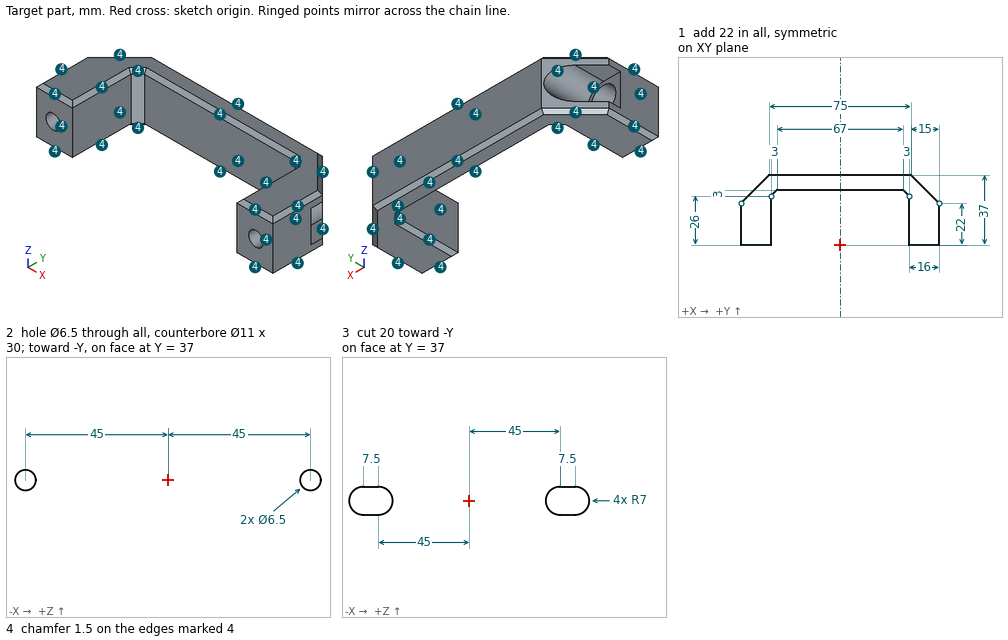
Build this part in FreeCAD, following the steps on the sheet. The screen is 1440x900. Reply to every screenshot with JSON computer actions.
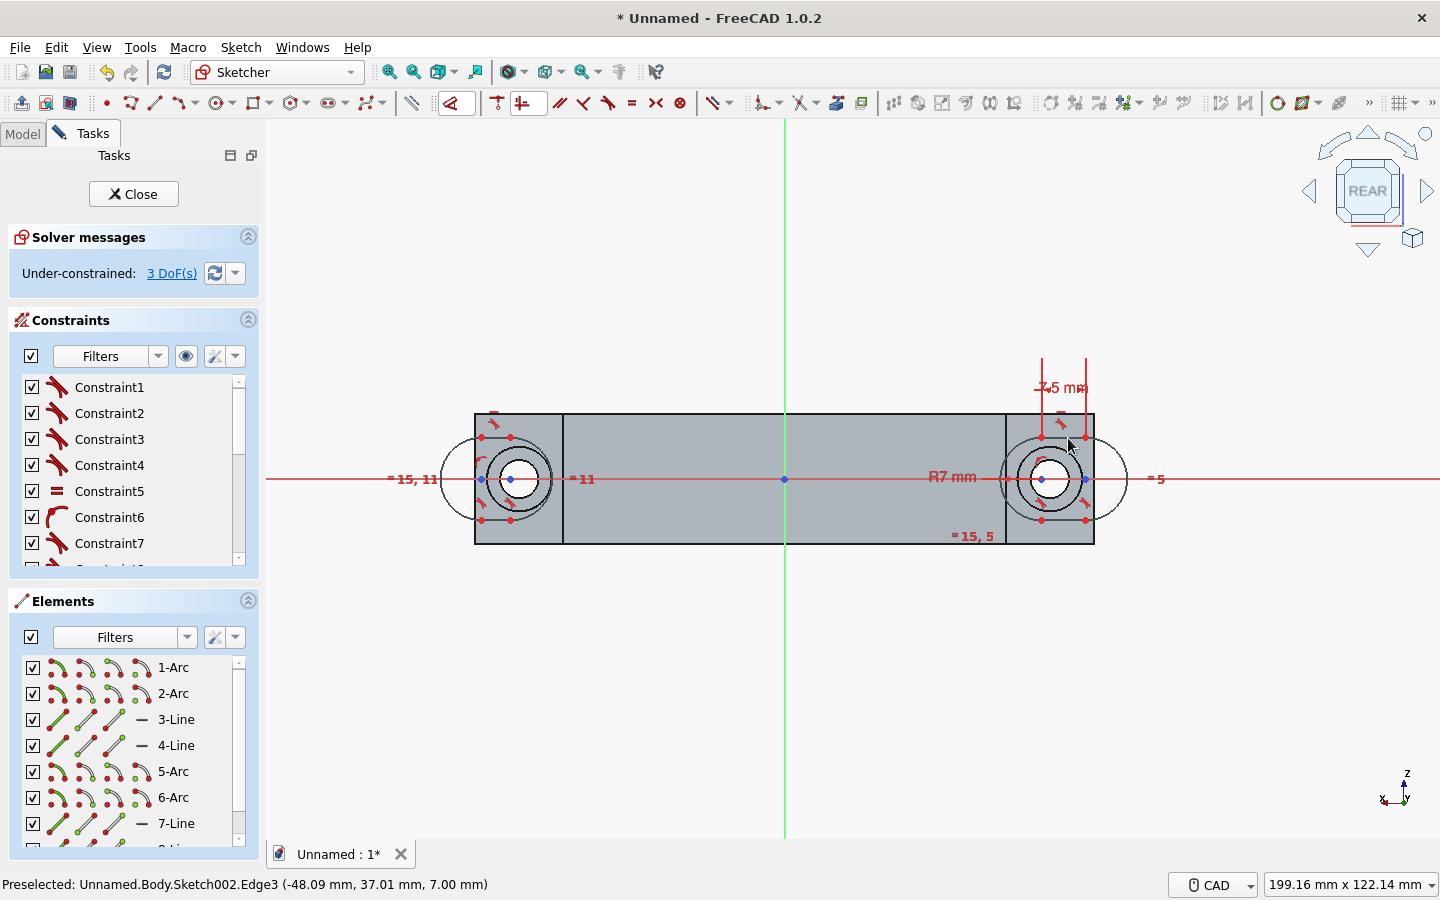
{"action": "left_click", "coordinate": [493, 438]}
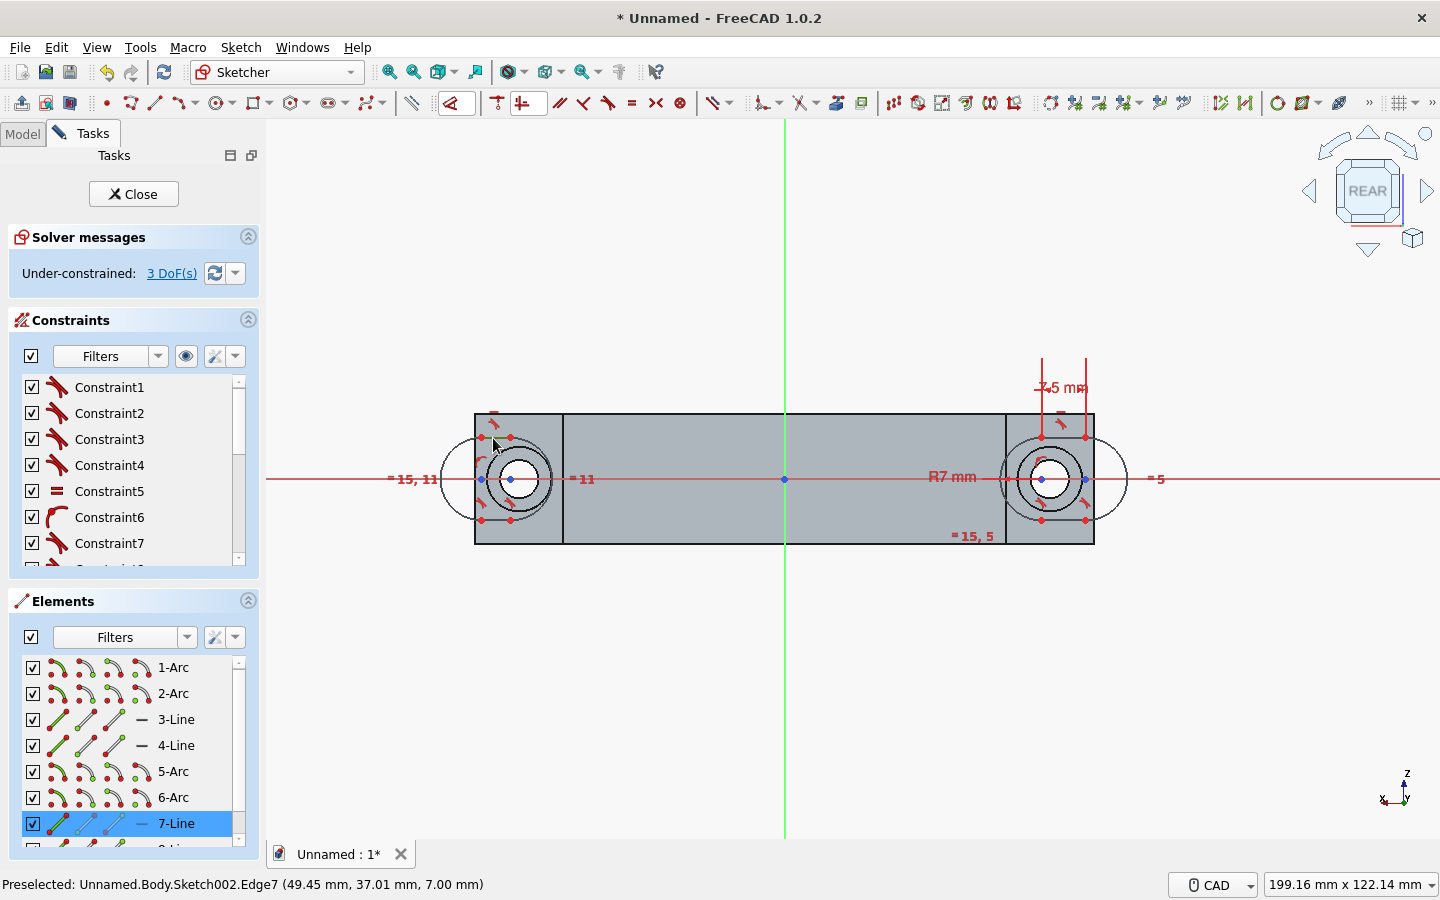
{"action": "left_click", "coordinate": [470, 104]}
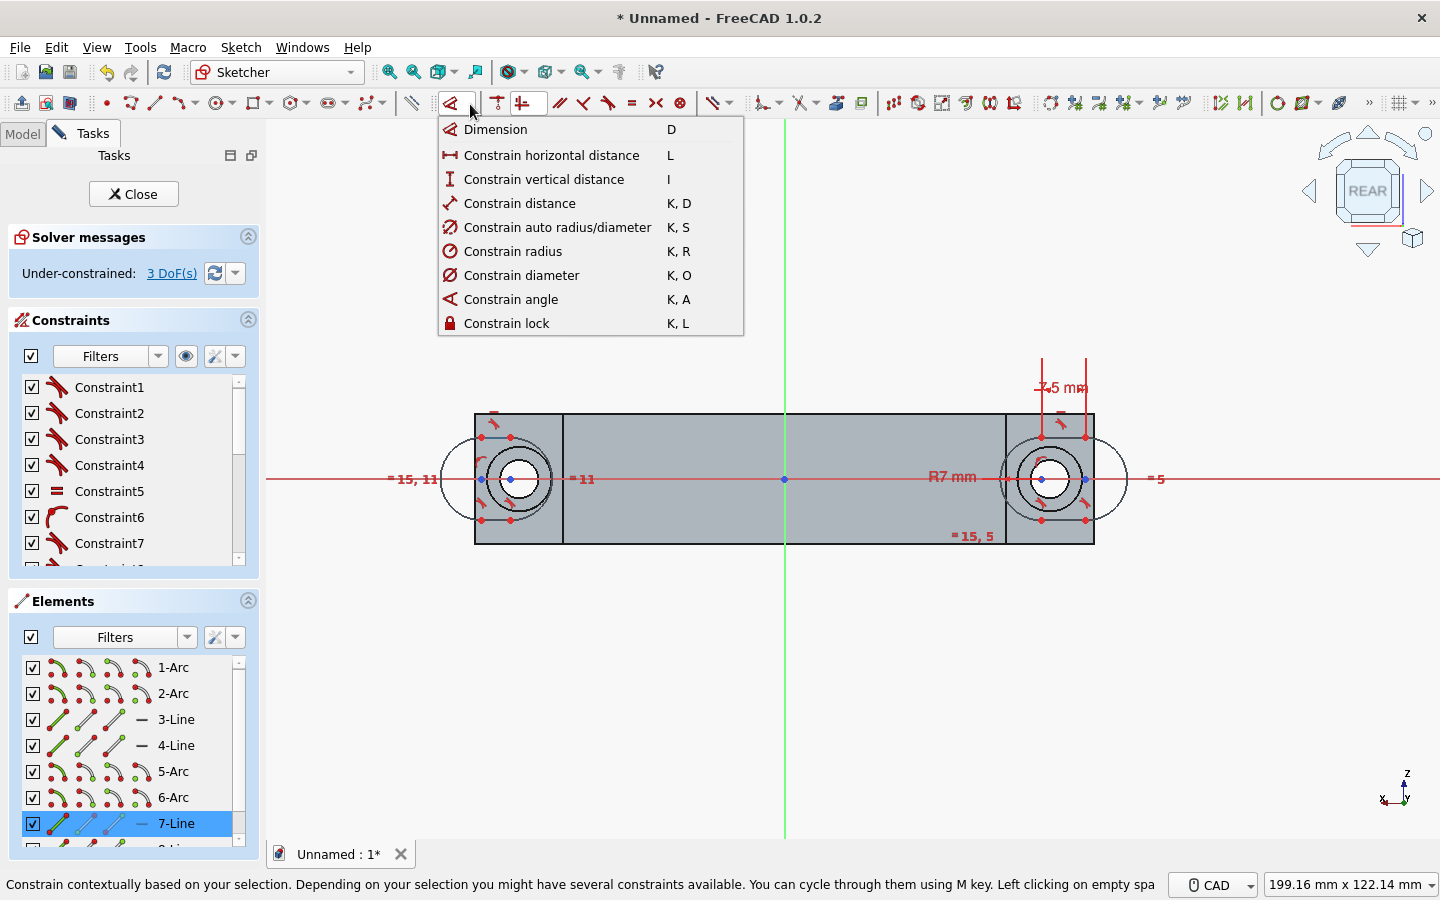
{"action": "left_click", "coordinate": [591, 155]}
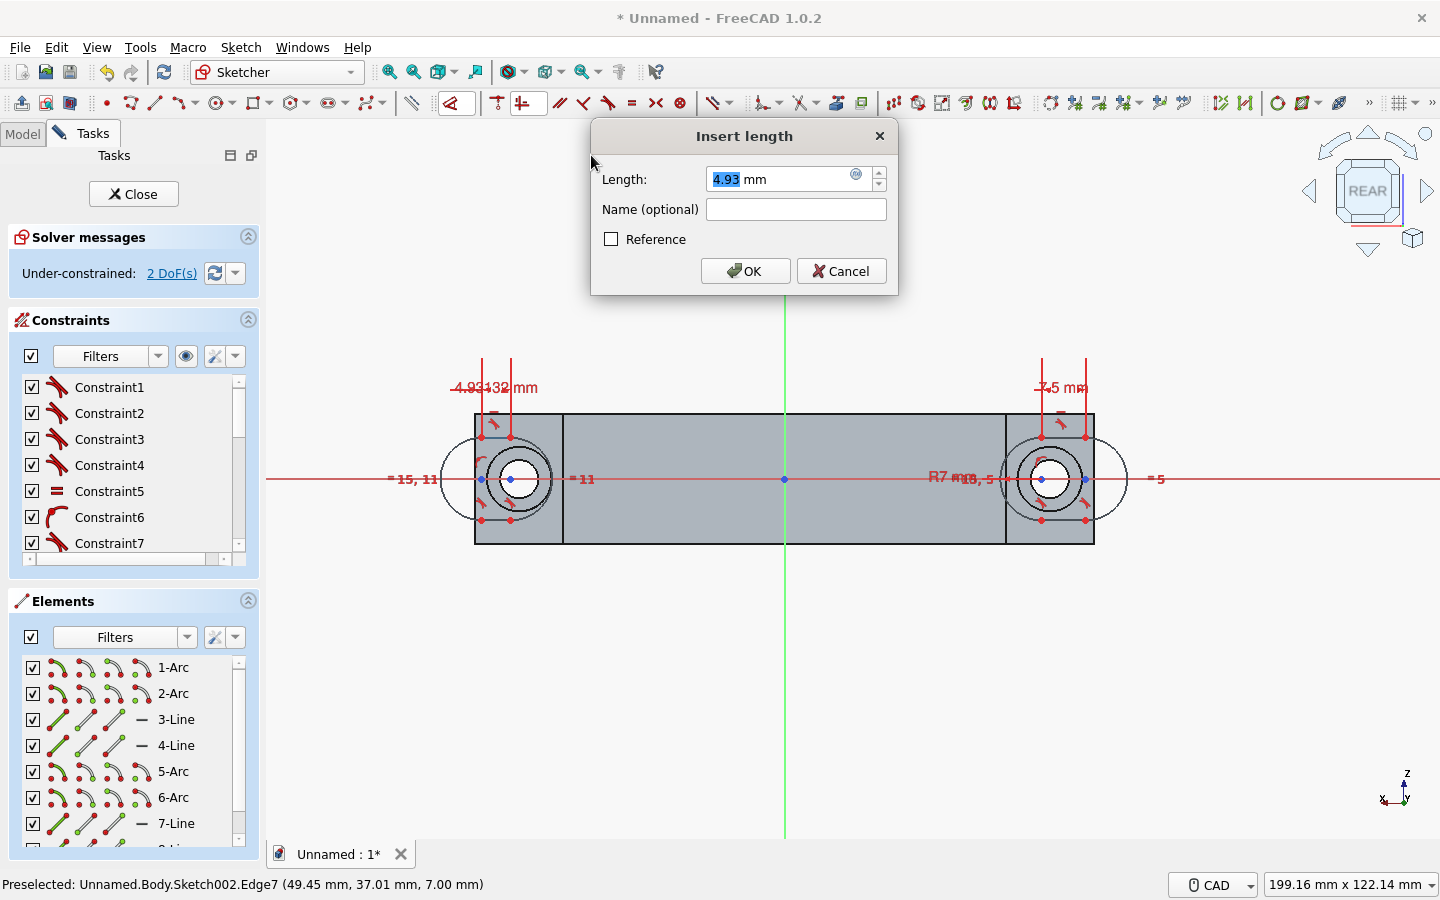
{"action": "type", "text": "7.5"}
{"action": "key", "text": "Return"}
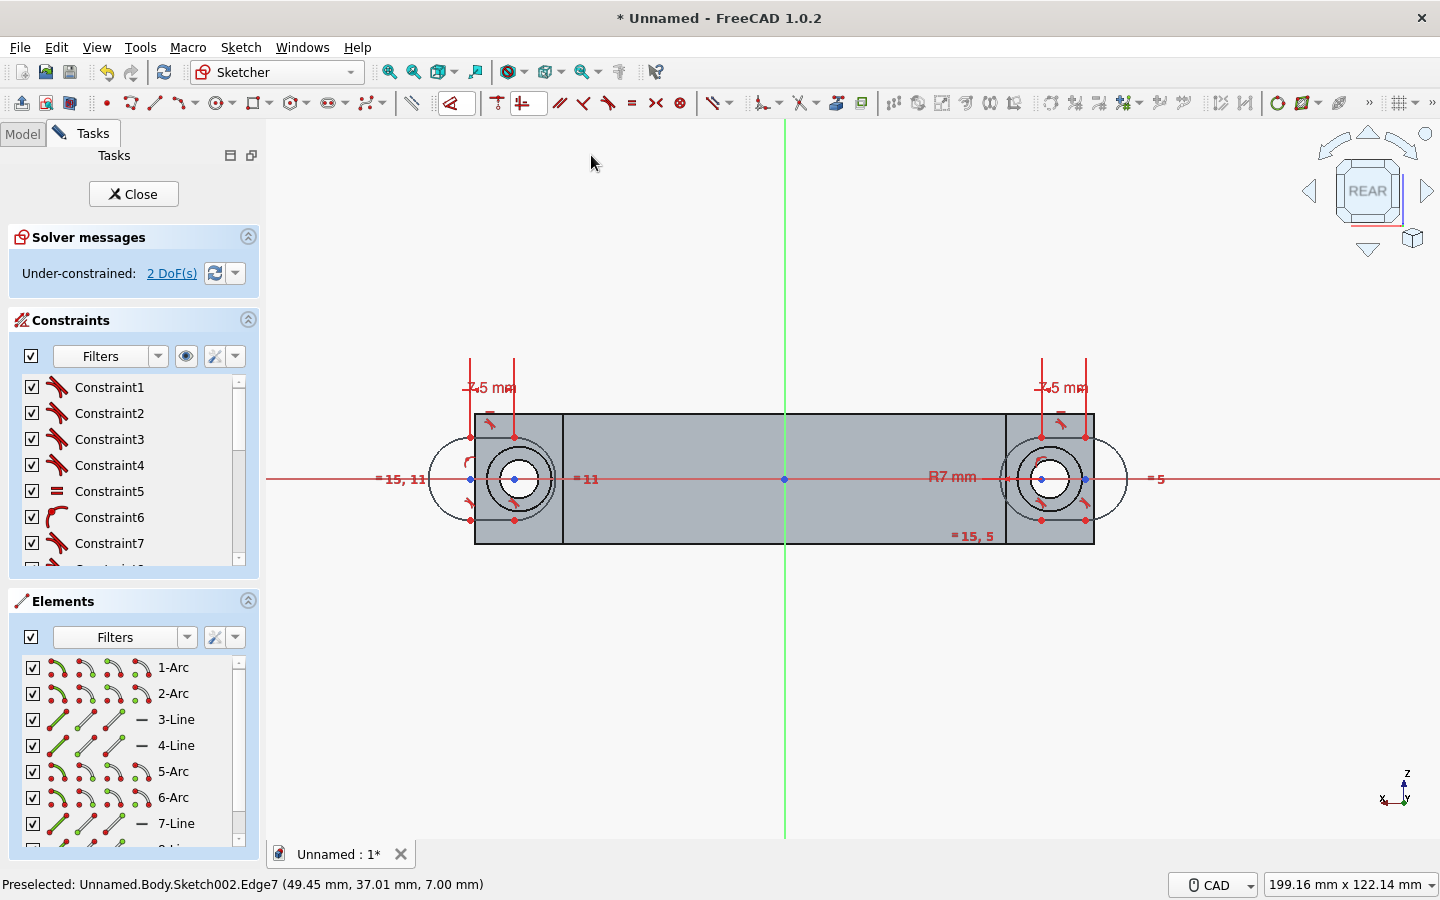
{"action": "left_click", "coordinate": [1042, 438]}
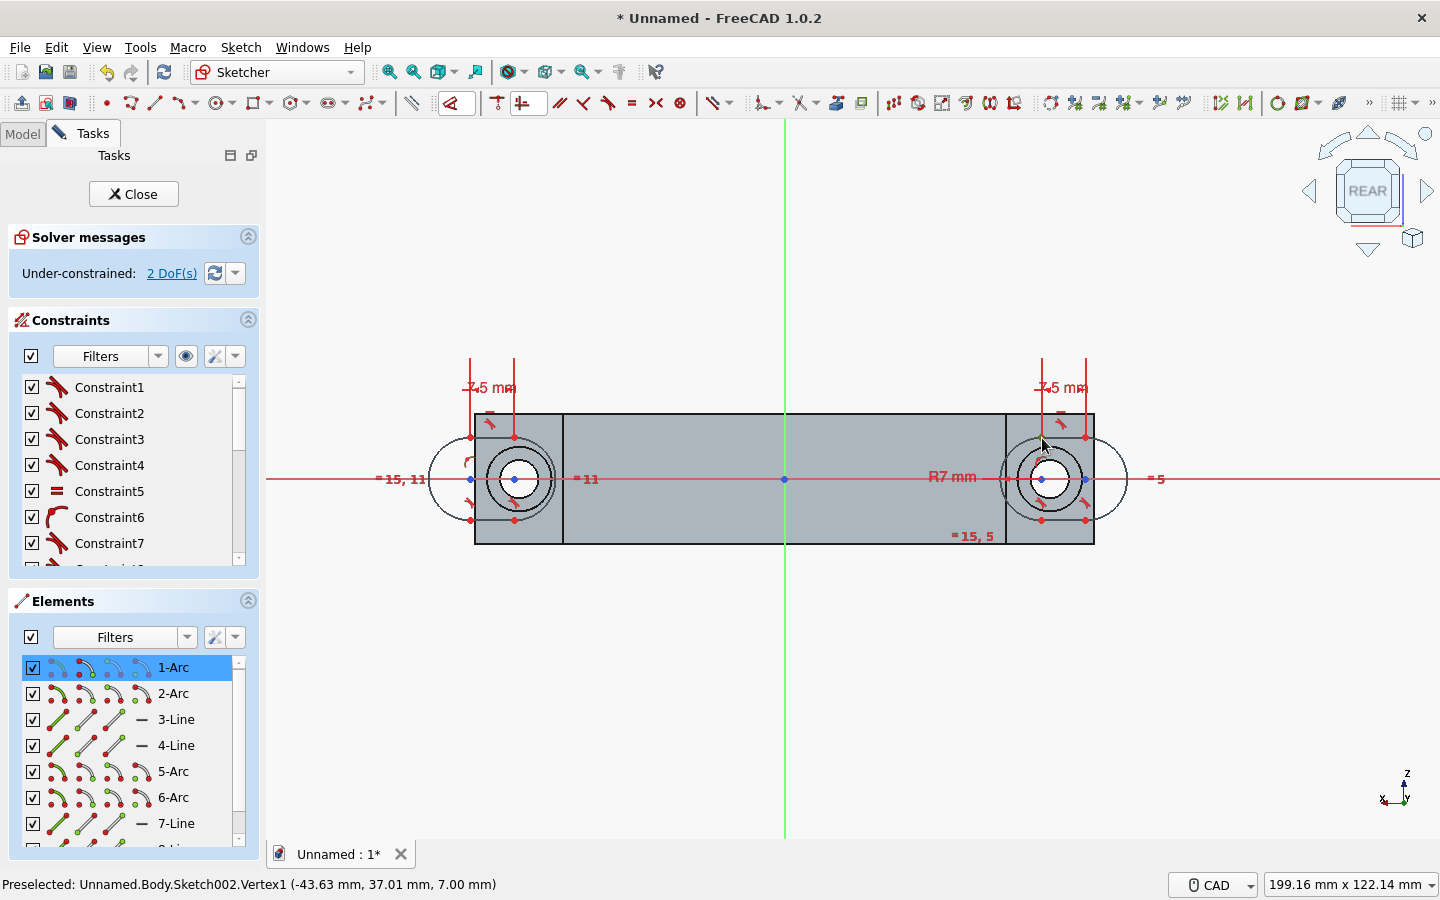
{"action": "left_click", "coordinate": [470, 104]}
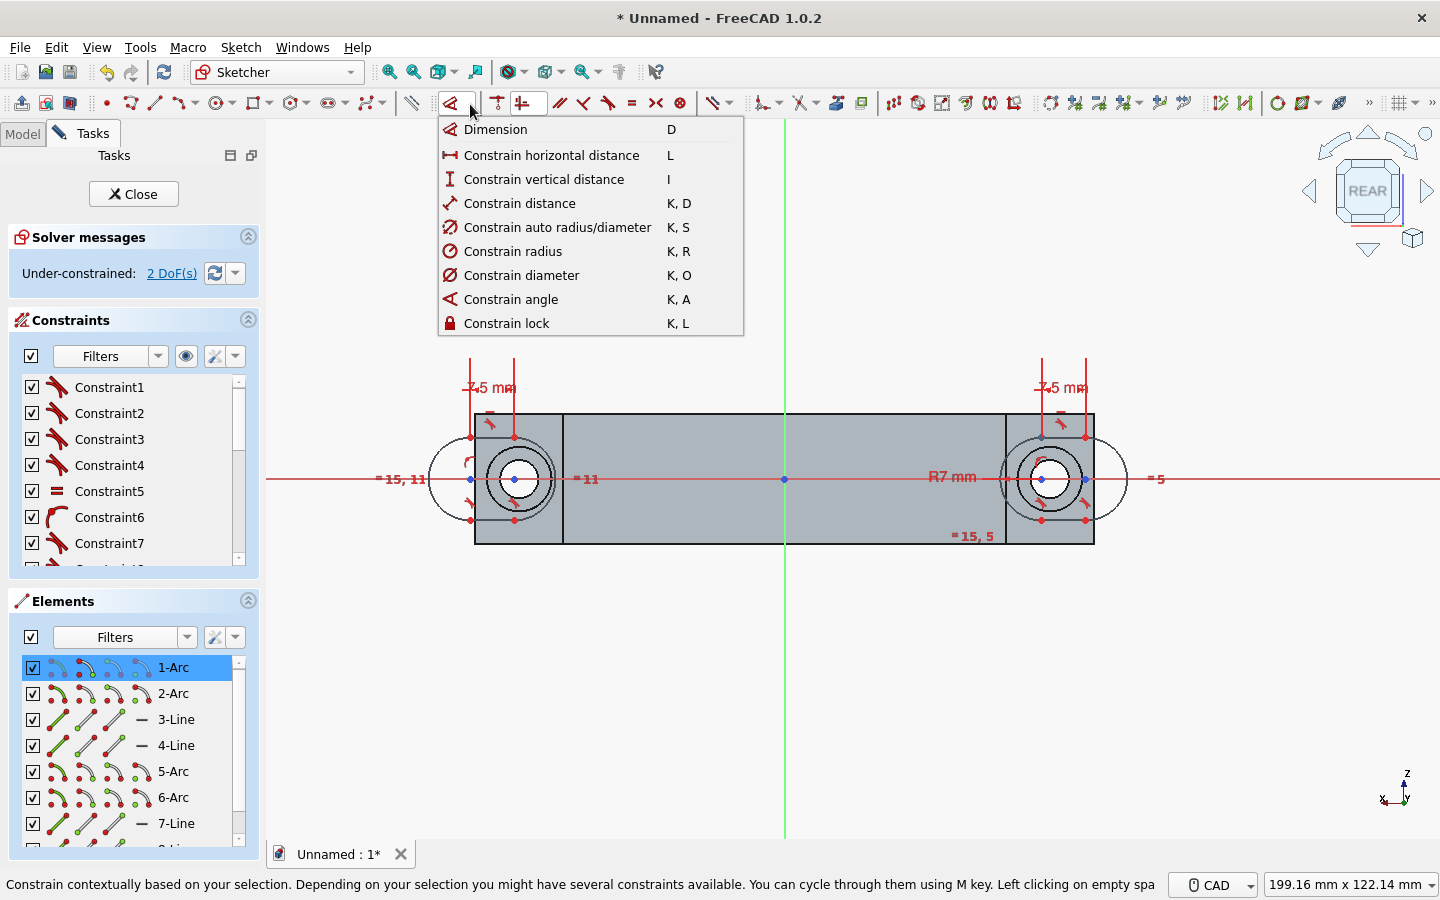
{"action": "left_click", "coordinate": [591, 155]}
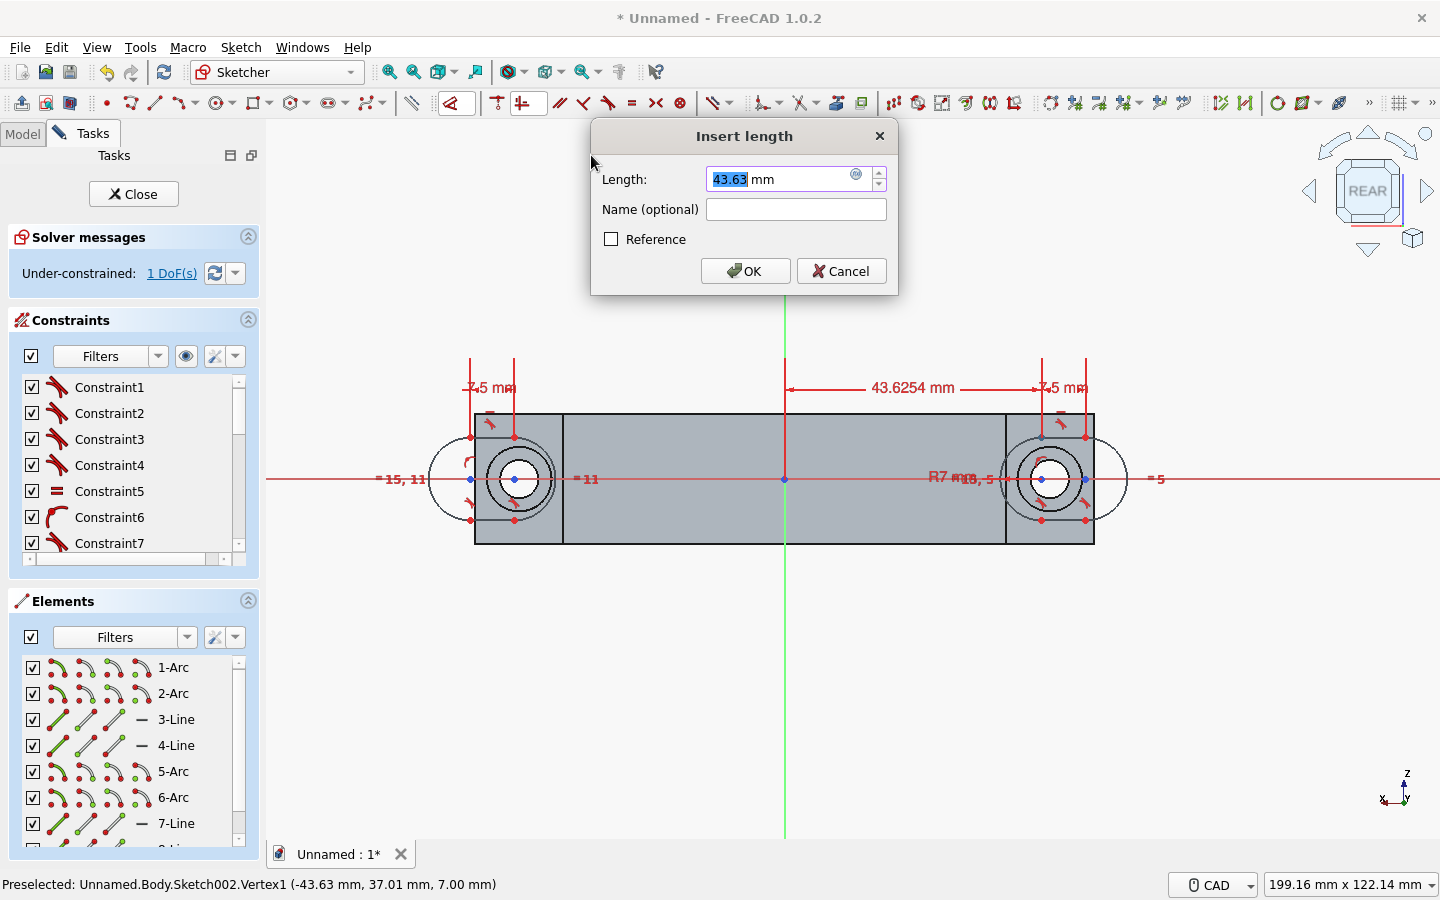
{"action": "type", "text": "45"}
{"action": "key", "text": "Return"}